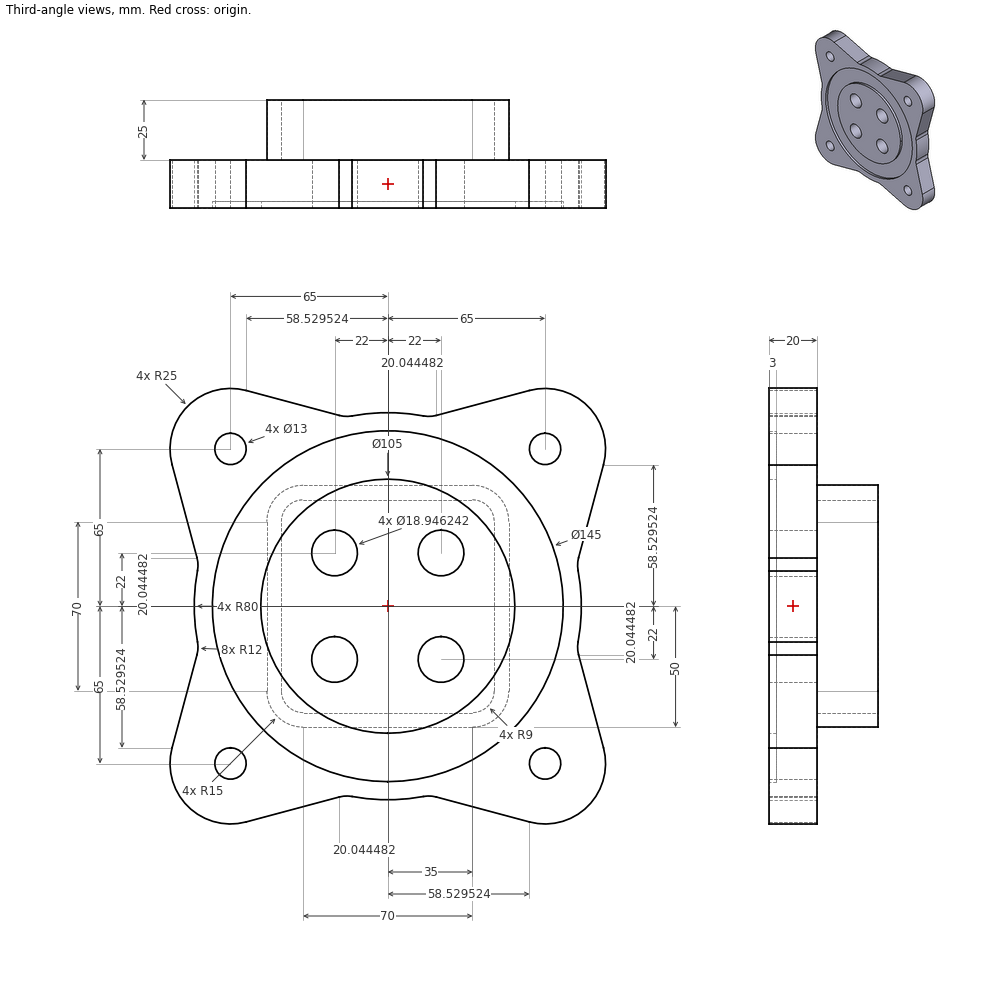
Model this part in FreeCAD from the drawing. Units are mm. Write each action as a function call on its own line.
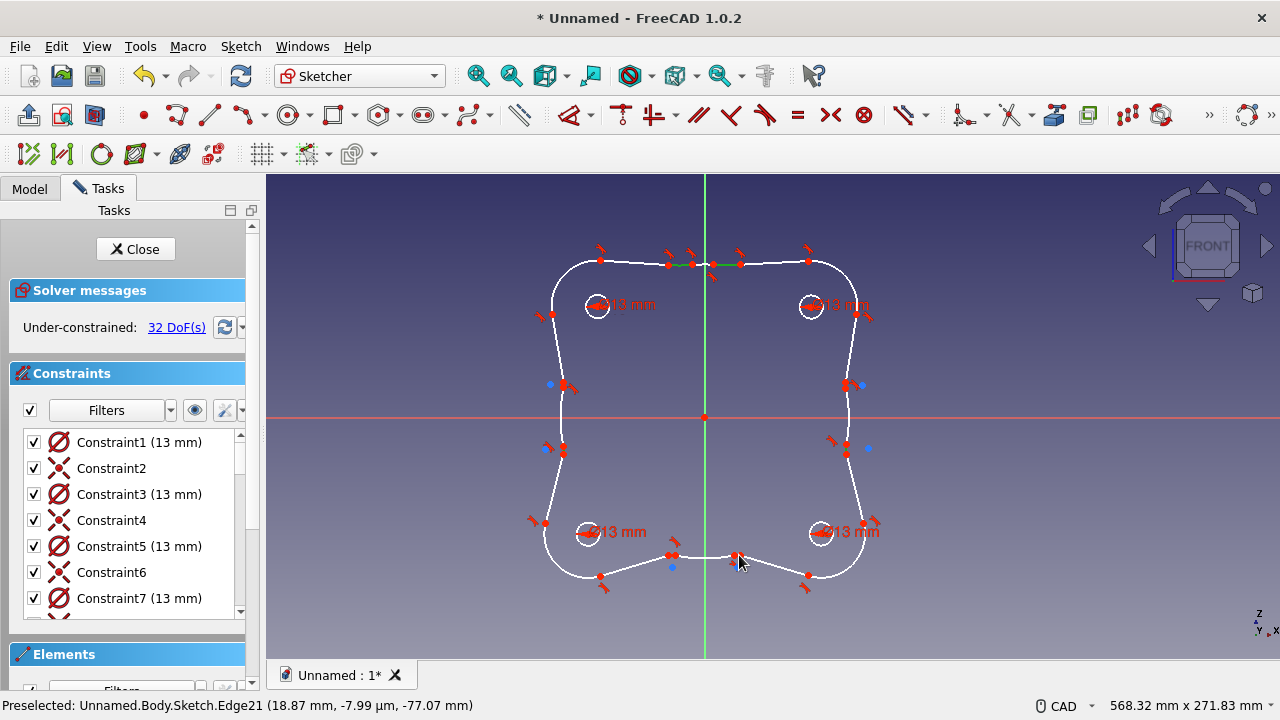
scroll(673, 555, up, 10)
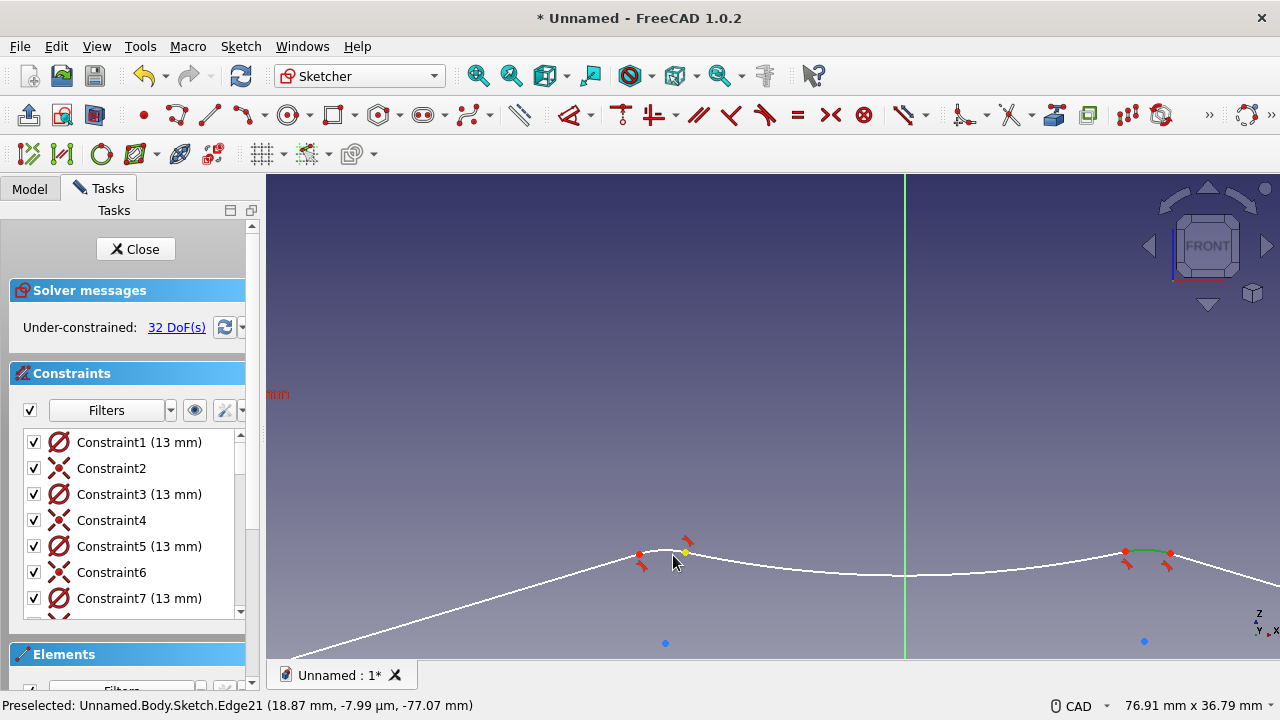
click(672, 550)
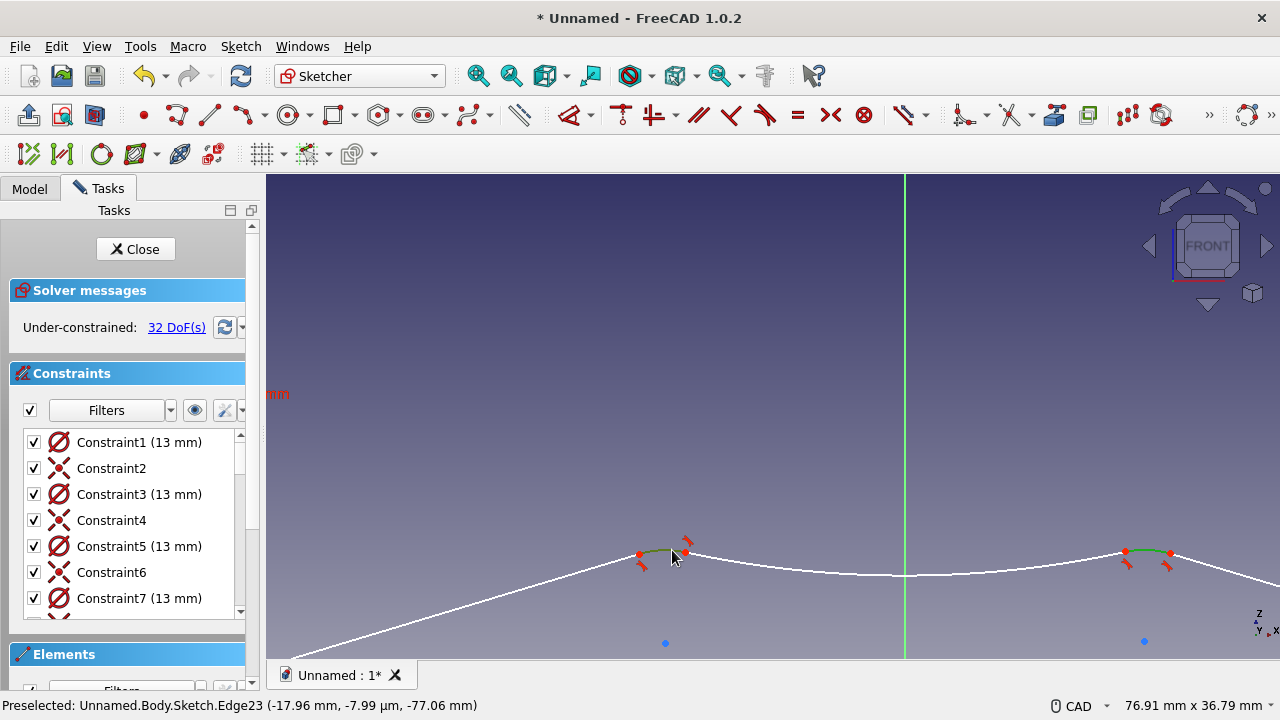
click(798, 116)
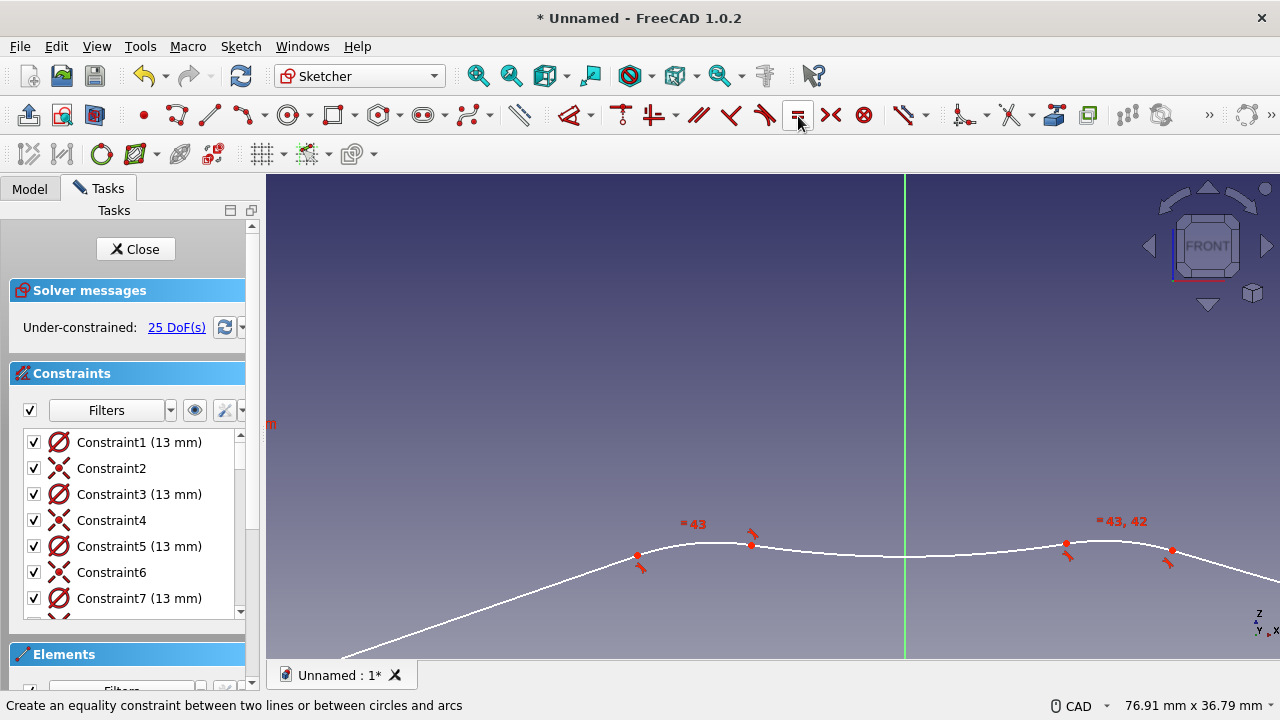
scroll(673, 555, down, 10)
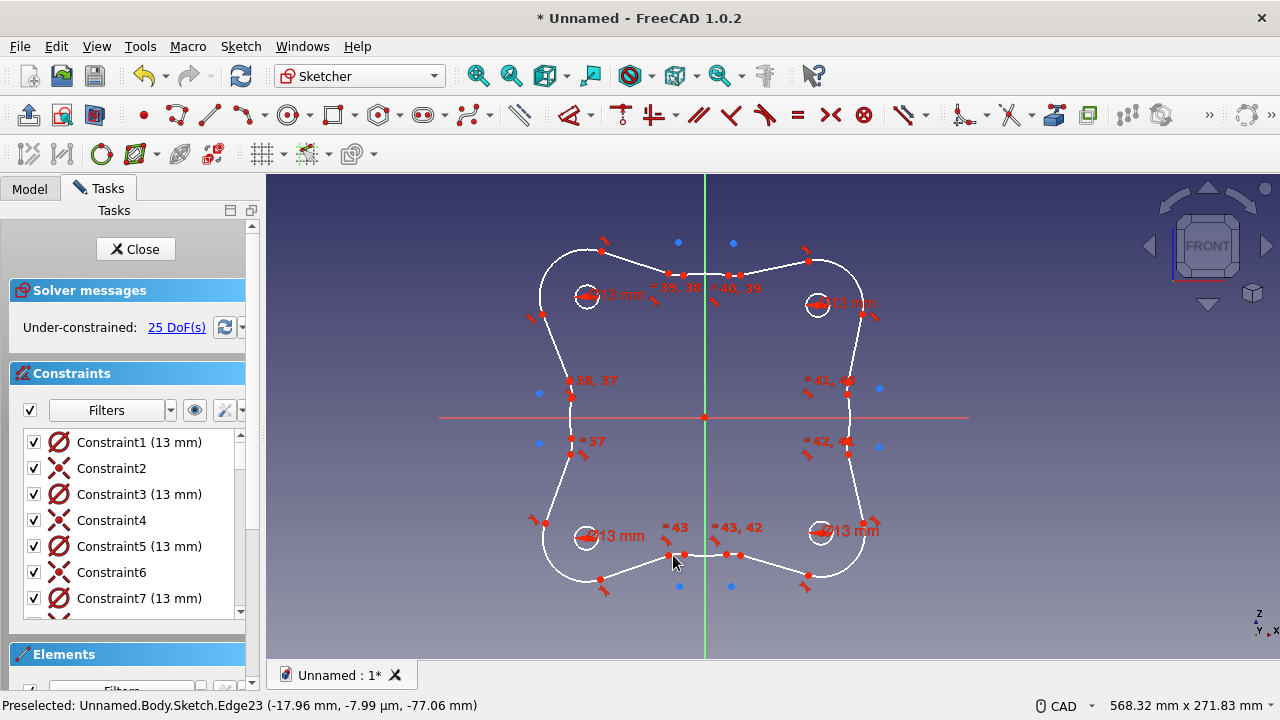
scroll(570, 410, up, 4)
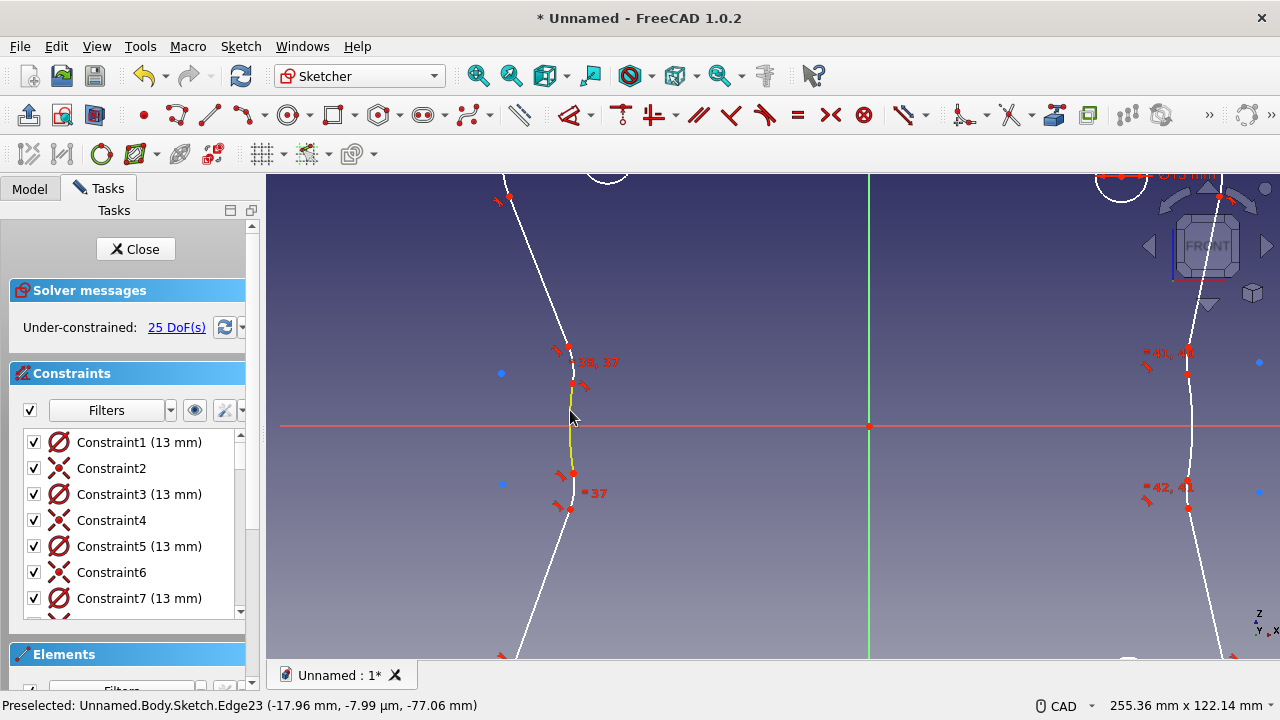
click(570, 410)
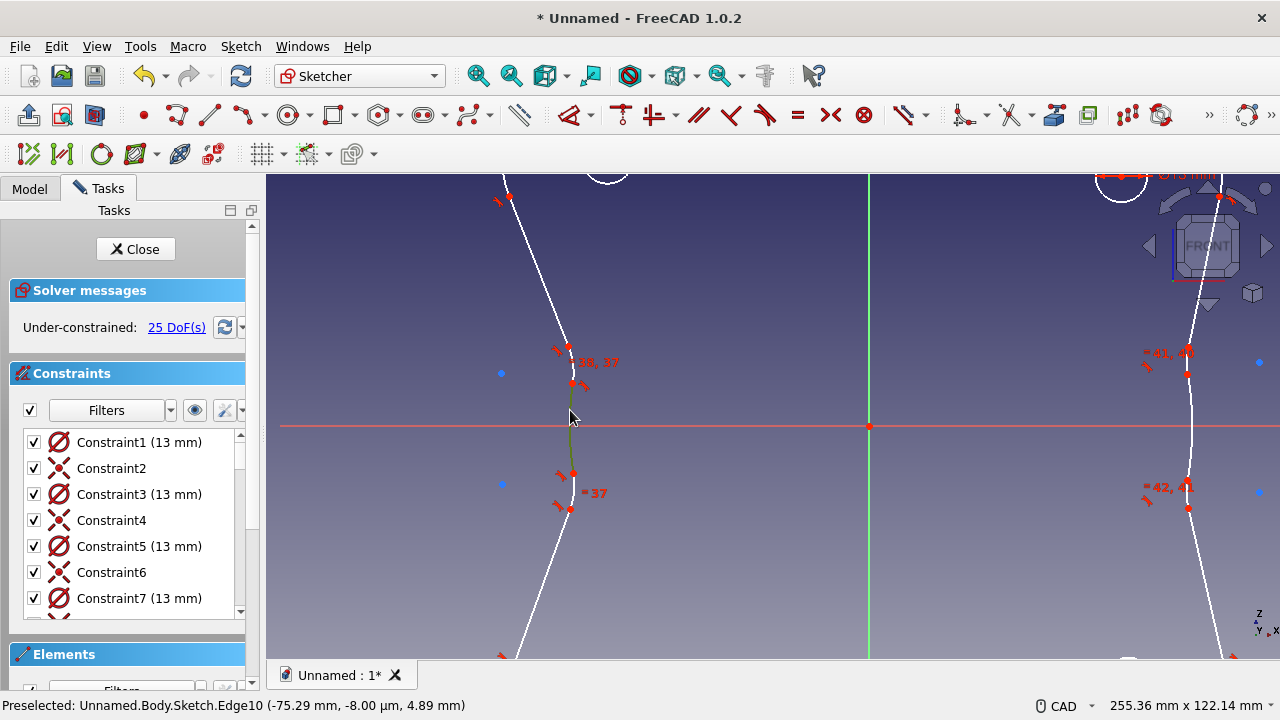
scroll(570, 409, down, 4)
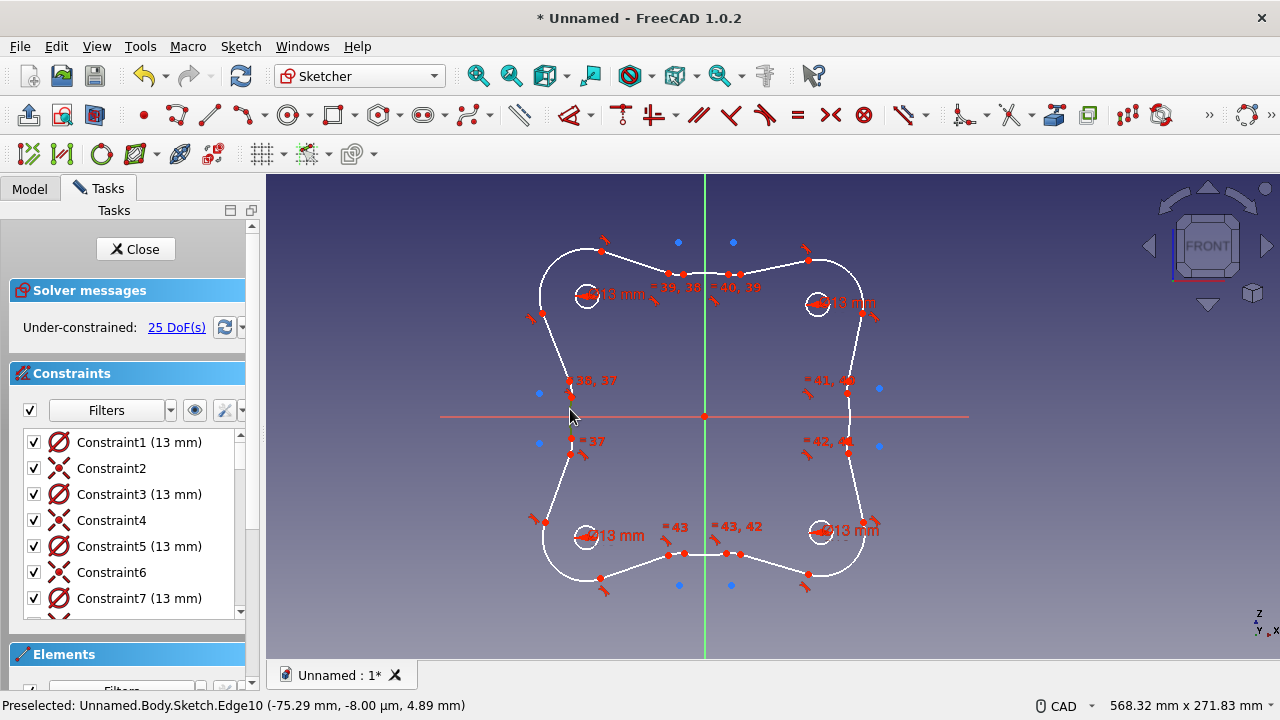
scroll(715, 273, up, 2)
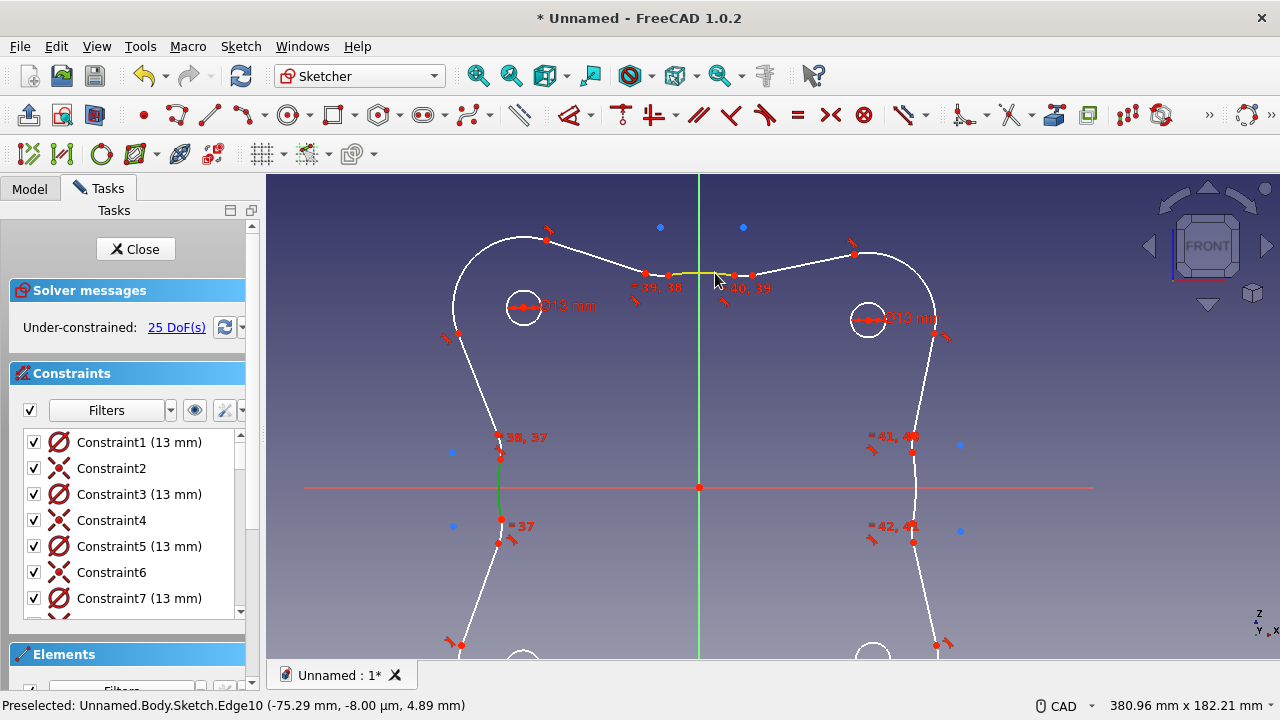
click(715, 273)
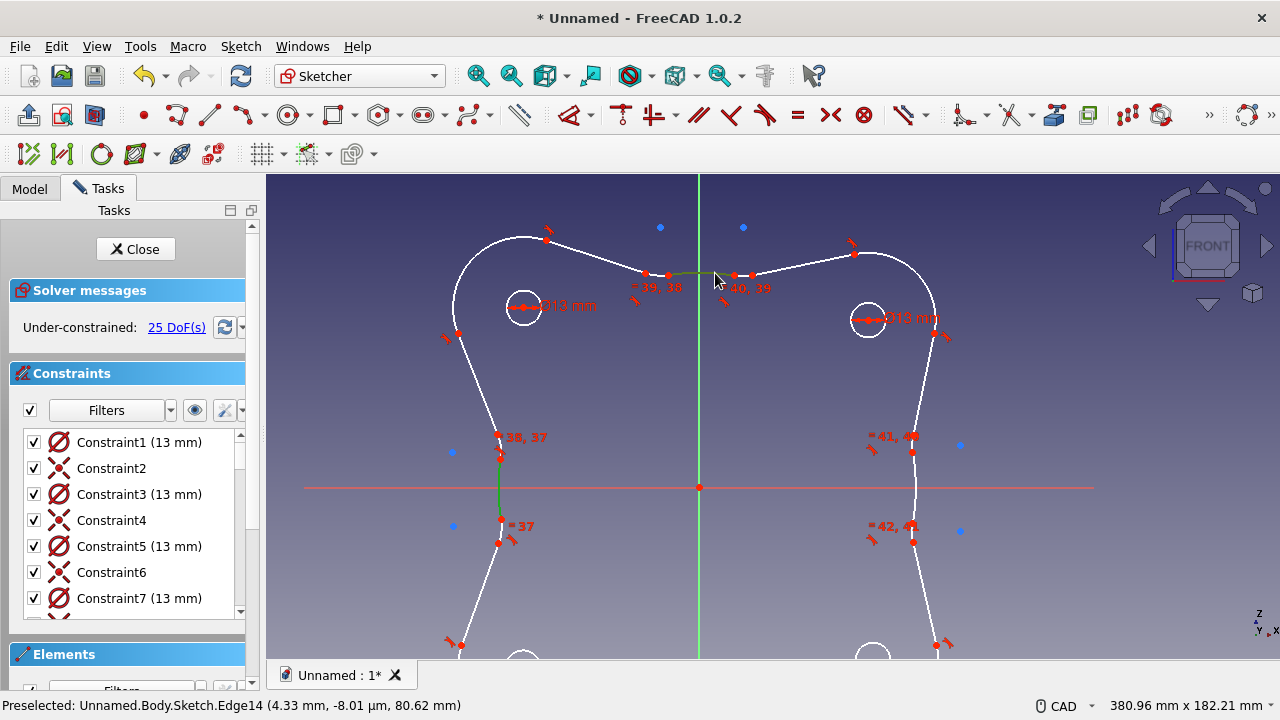
click(915, 503)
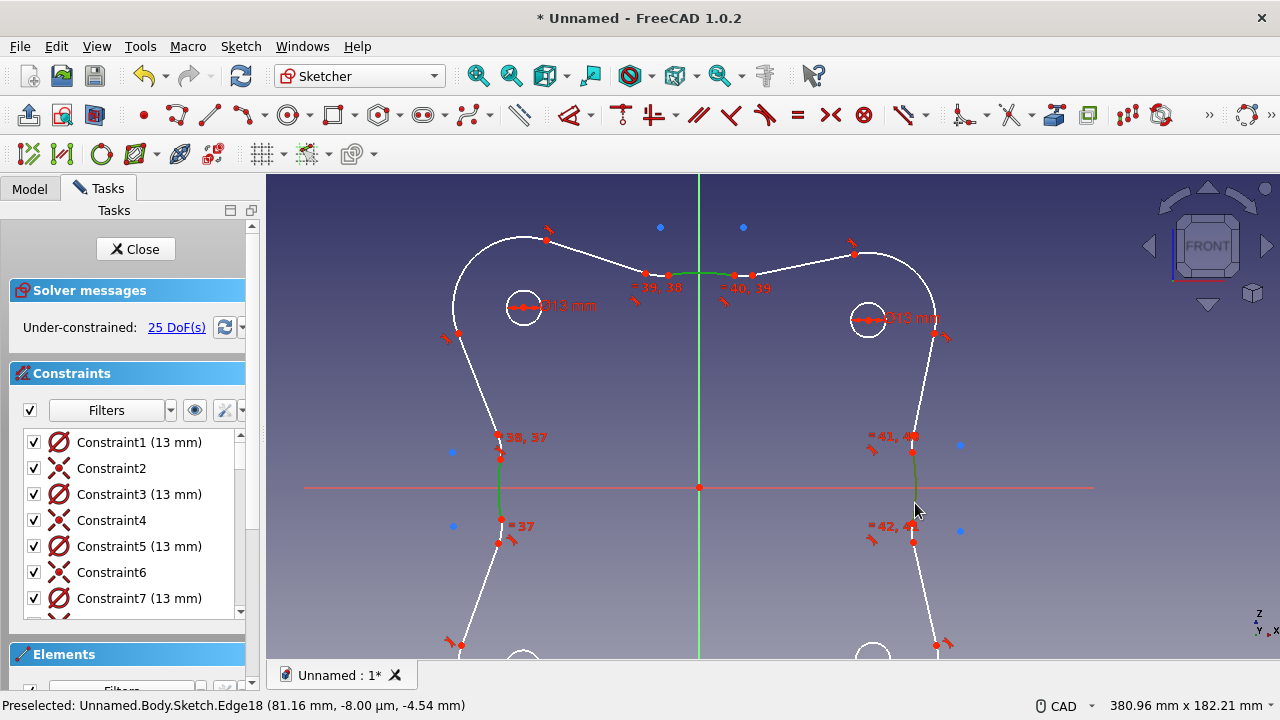
scroll(715, 272, down, 2)